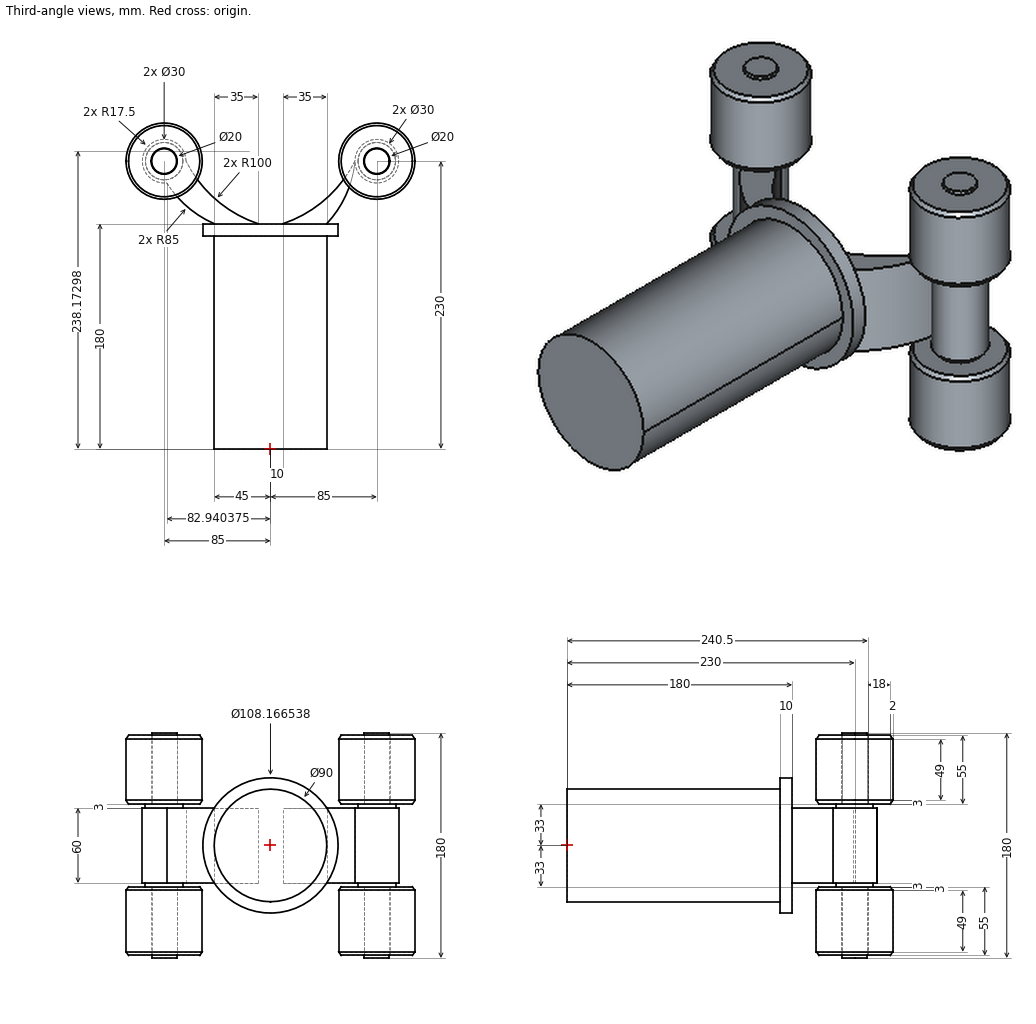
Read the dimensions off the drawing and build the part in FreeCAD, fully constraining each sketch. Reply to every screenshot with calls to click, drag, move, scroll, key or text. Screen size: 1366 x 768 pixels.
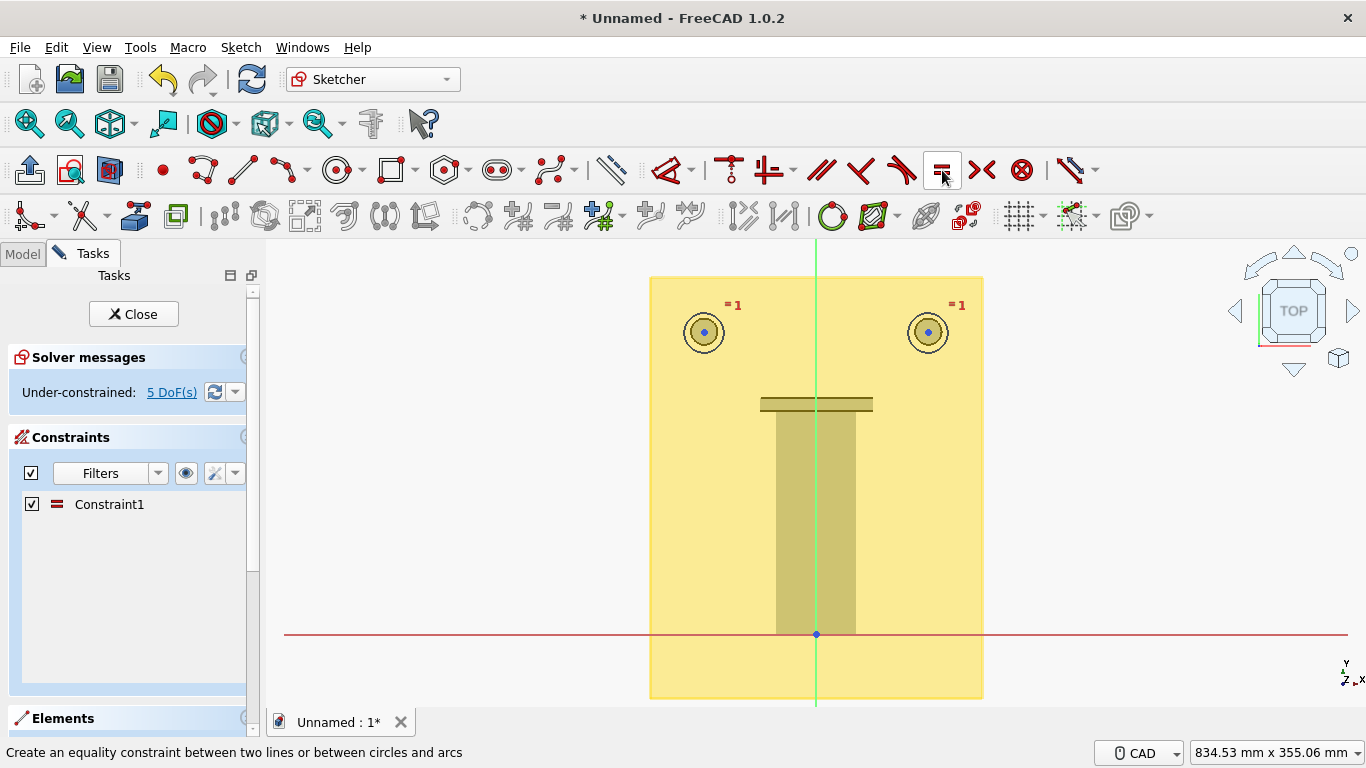
click(666, 170)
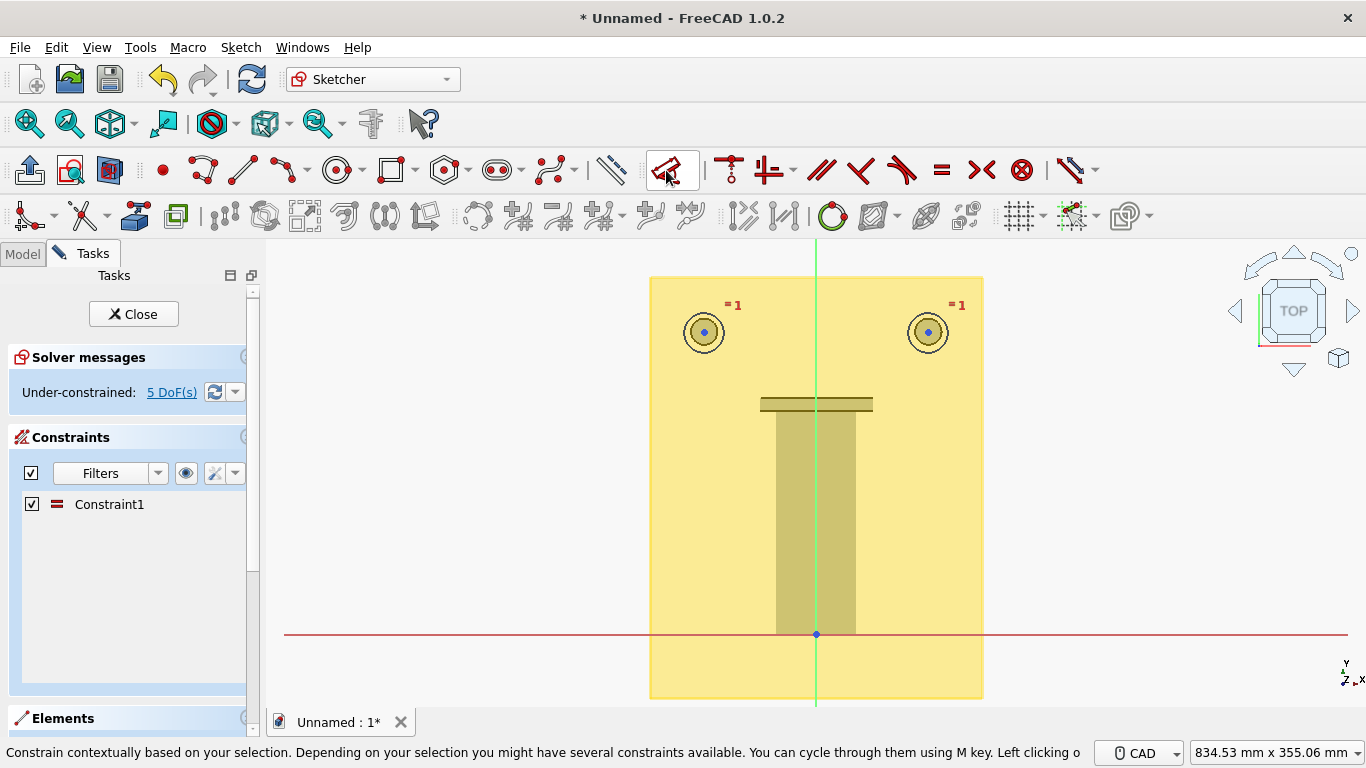
click(942, 319)
click(965, 296)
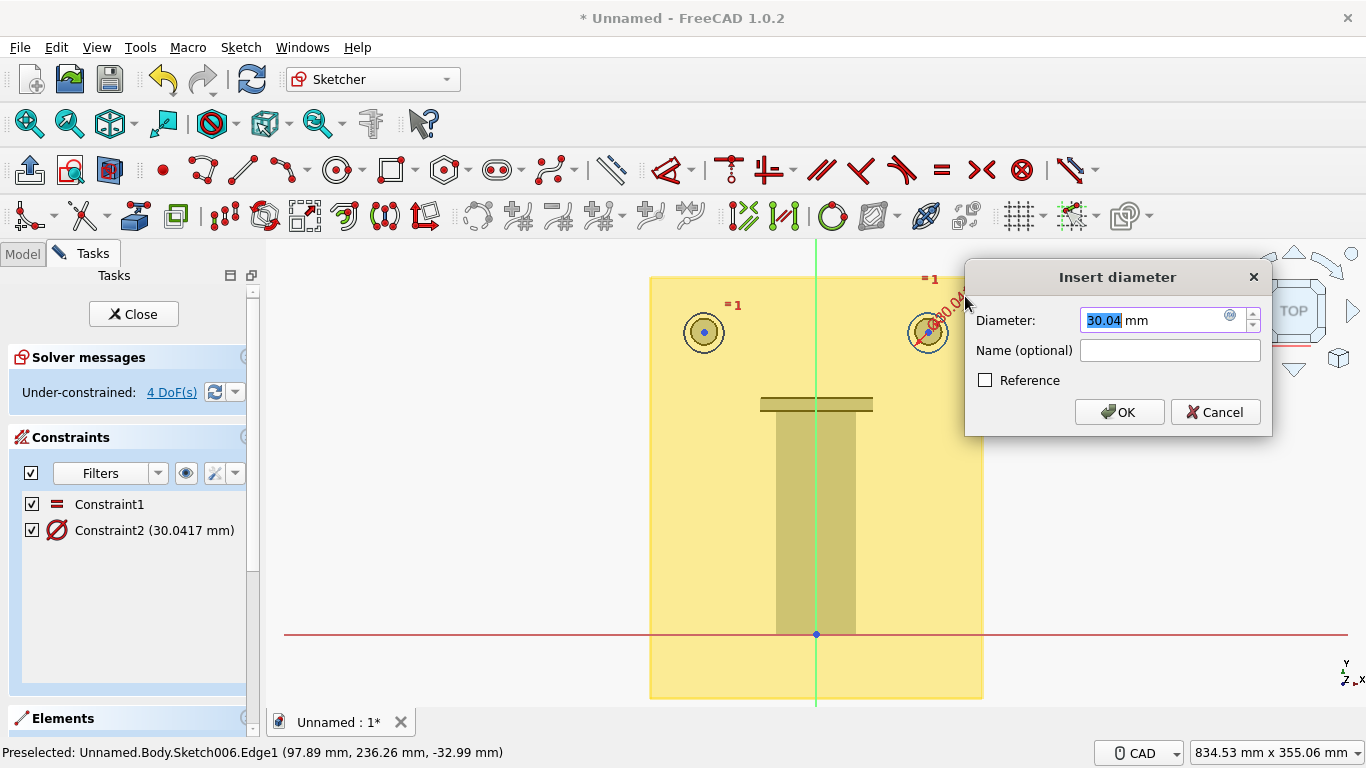
text(30)
key(Return)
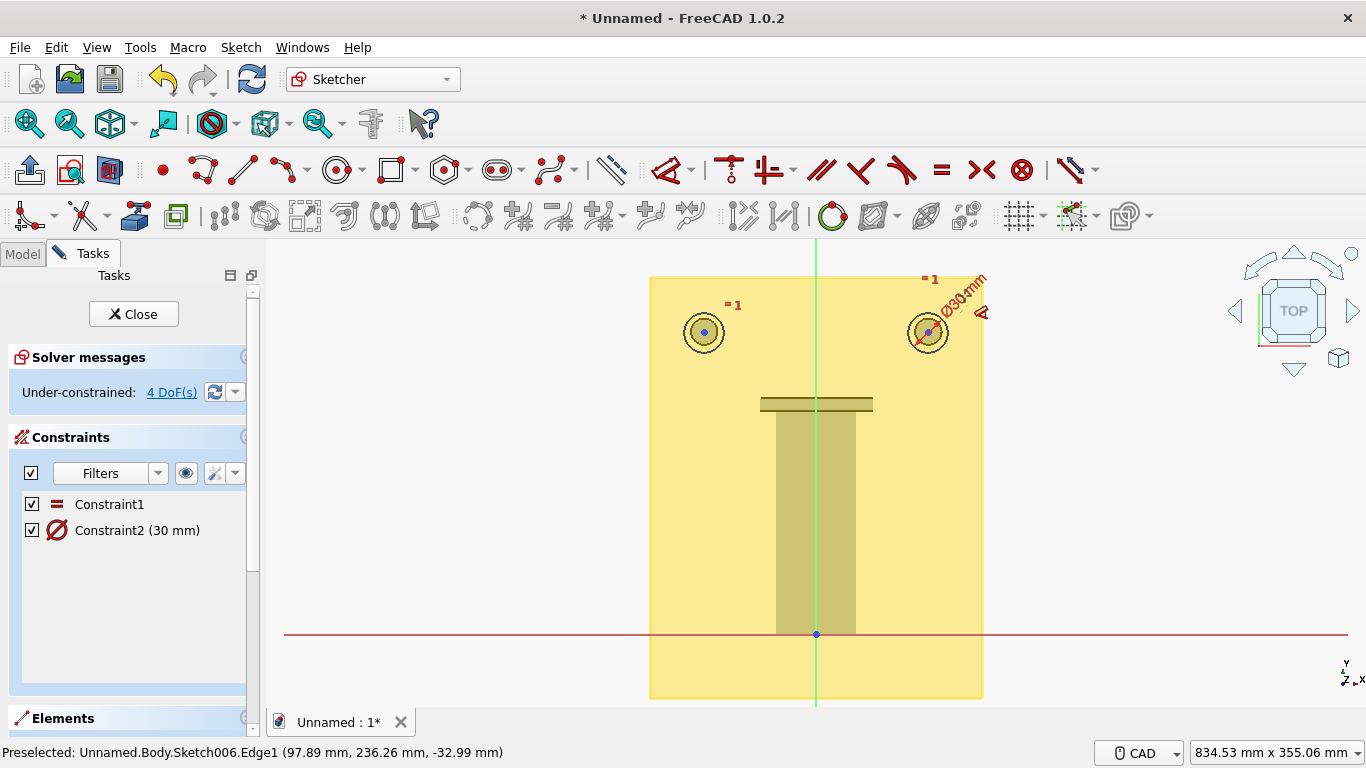
click(928, 333)
click(872, 669)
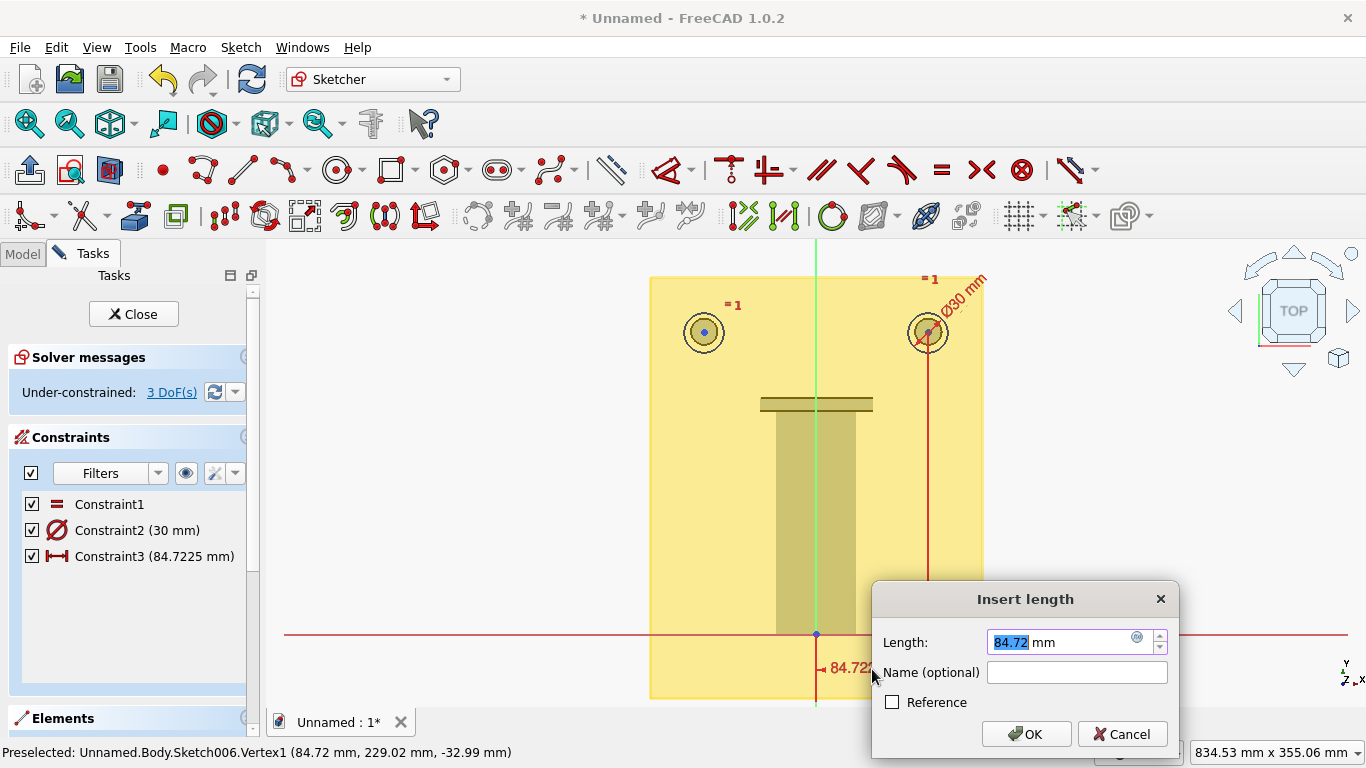
text(85)
key(Return)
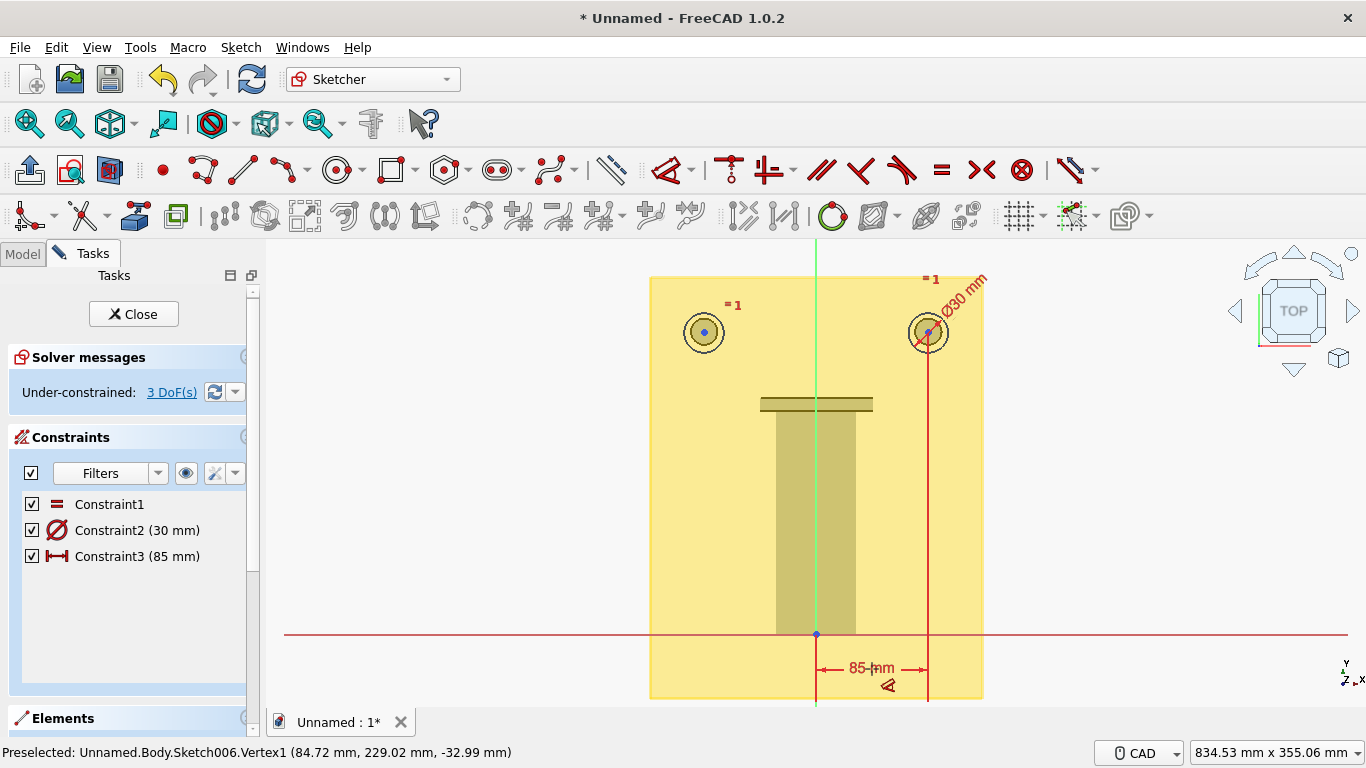
click(704, 333)
click(760, 669)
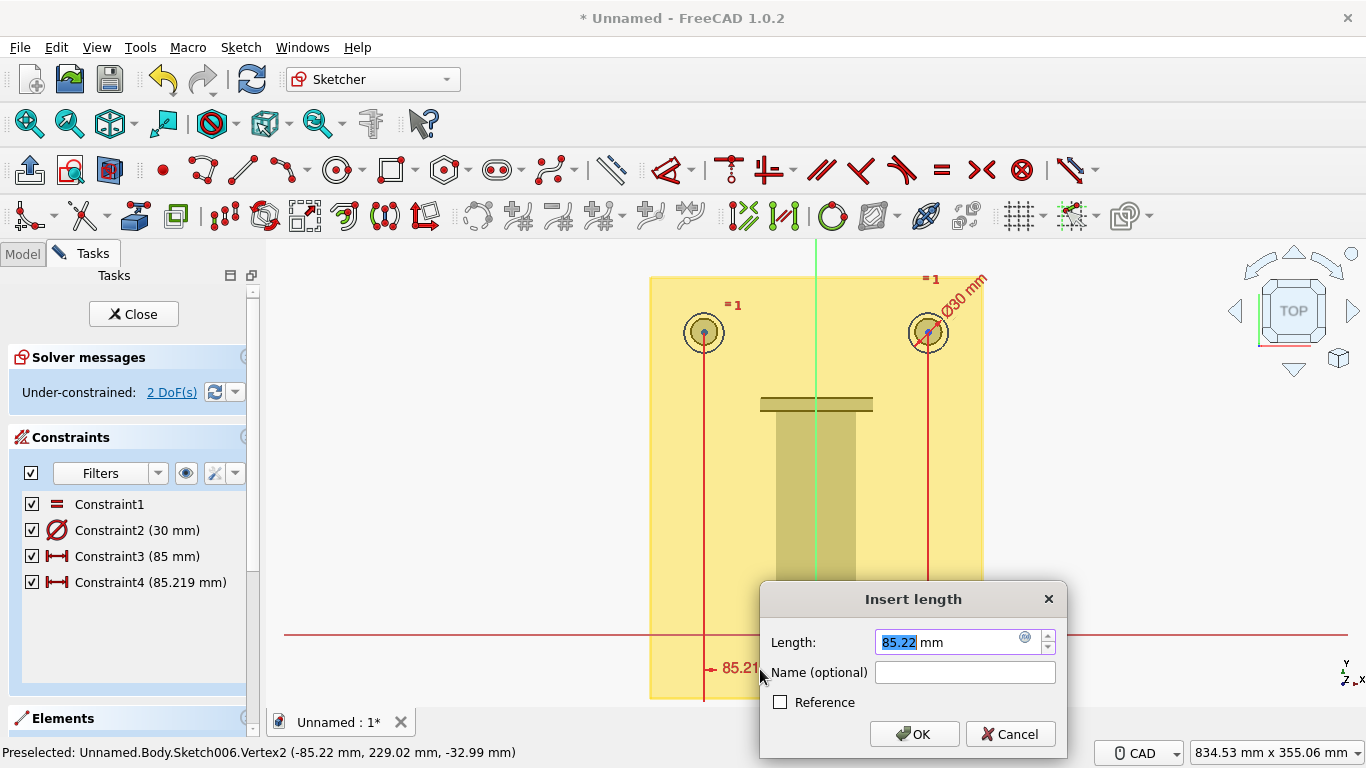
text(85)
key(Return)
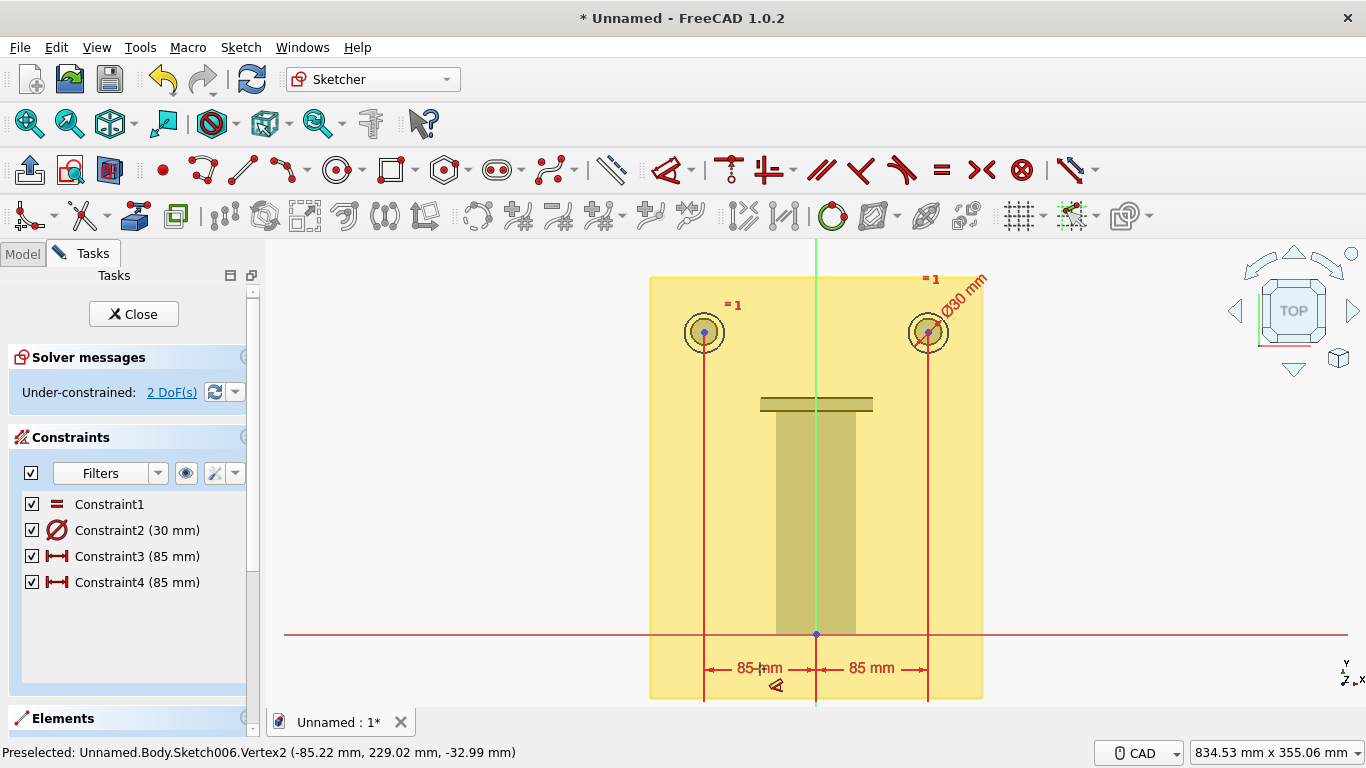
click(928, 333)
click(962, 484)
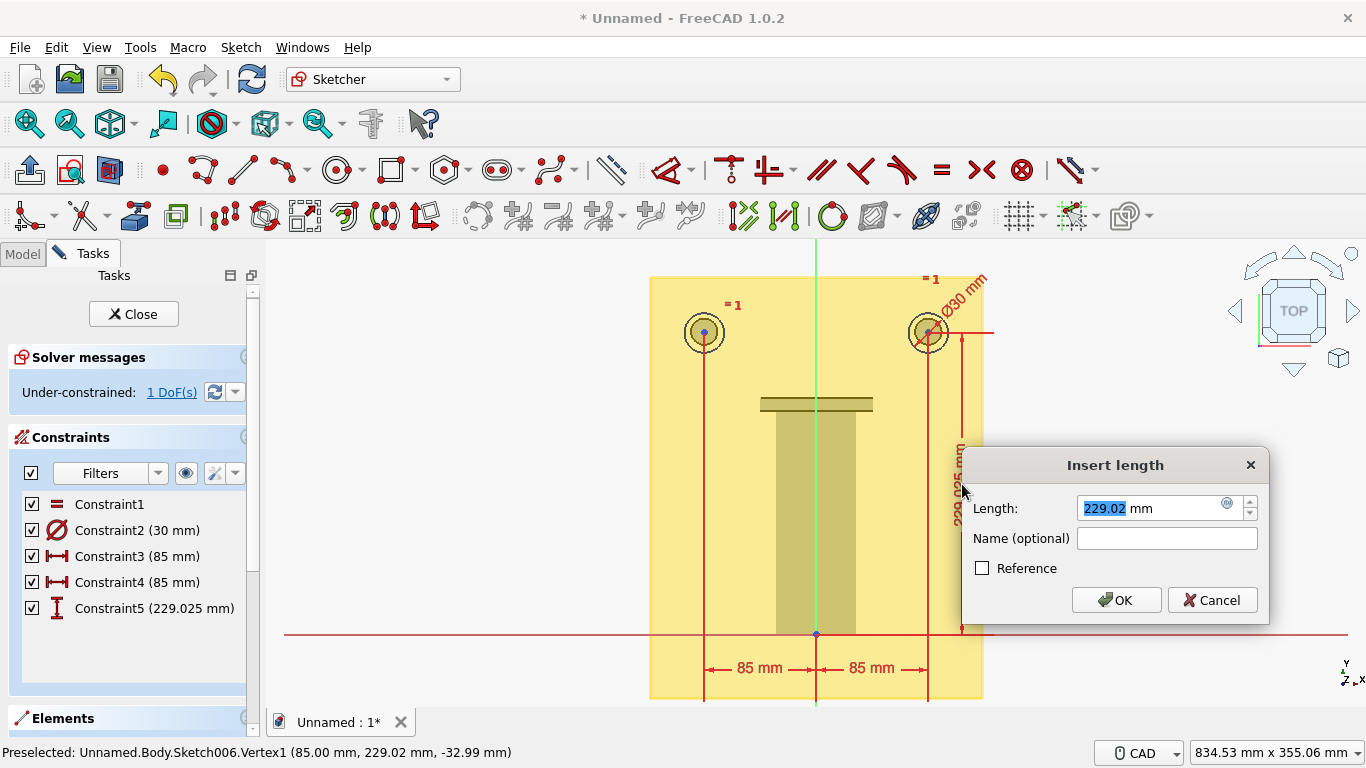
text(230)
key(Return)